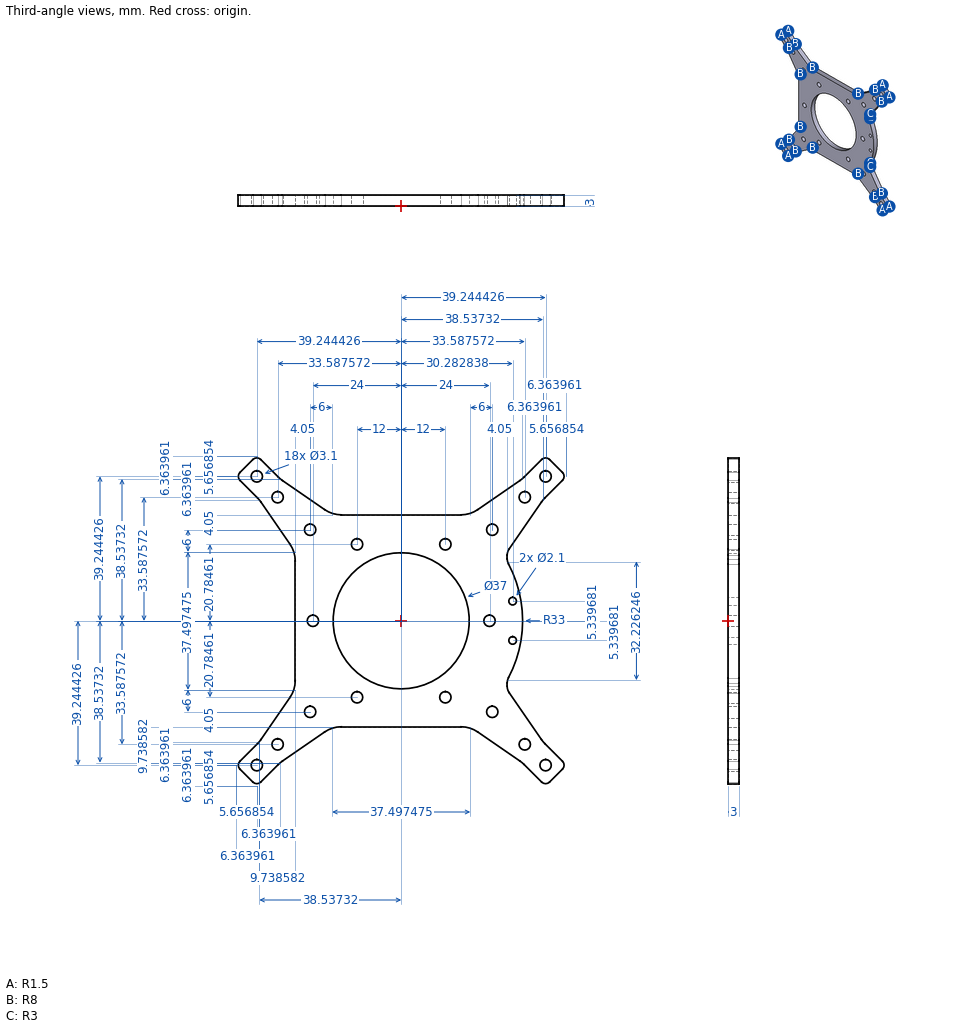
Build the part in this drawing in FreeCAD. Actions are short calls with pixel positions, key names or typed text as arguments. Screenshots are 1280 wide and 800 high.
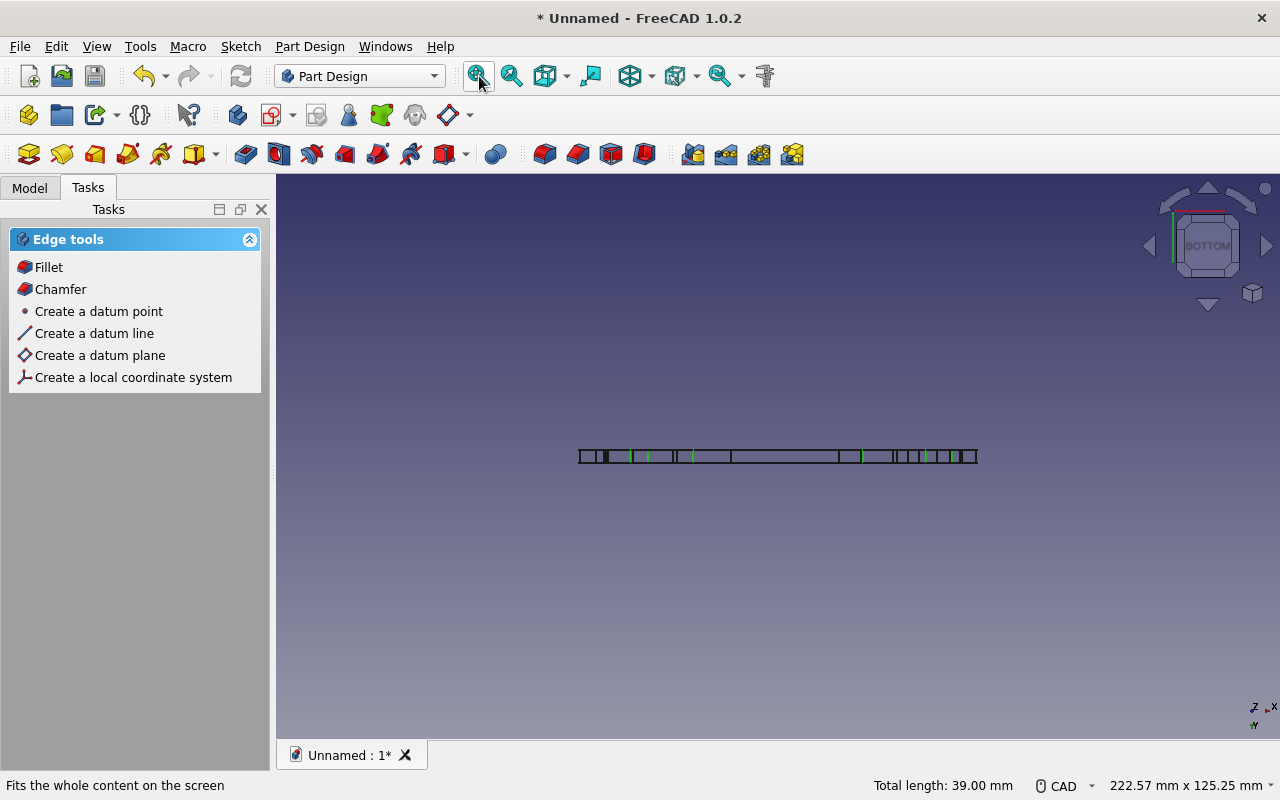
key(4)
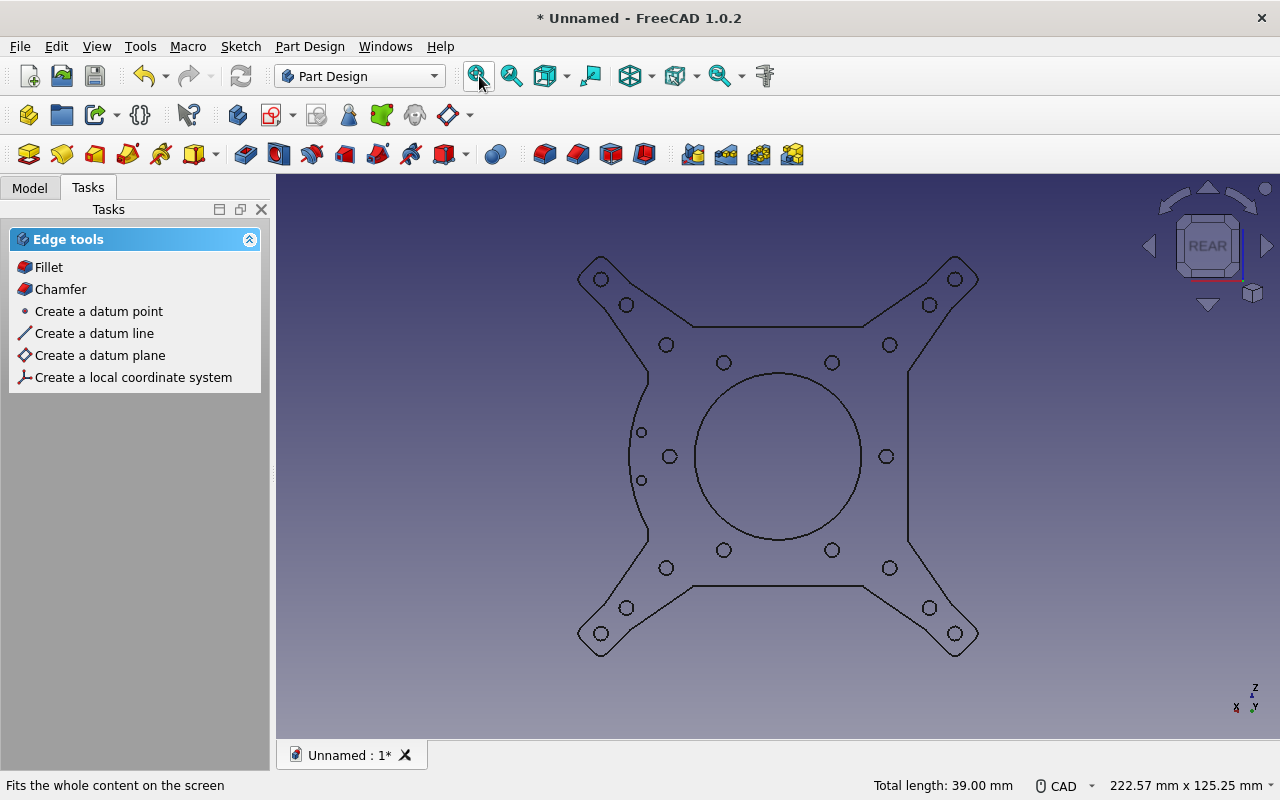
scroll(952, 604, up, 6)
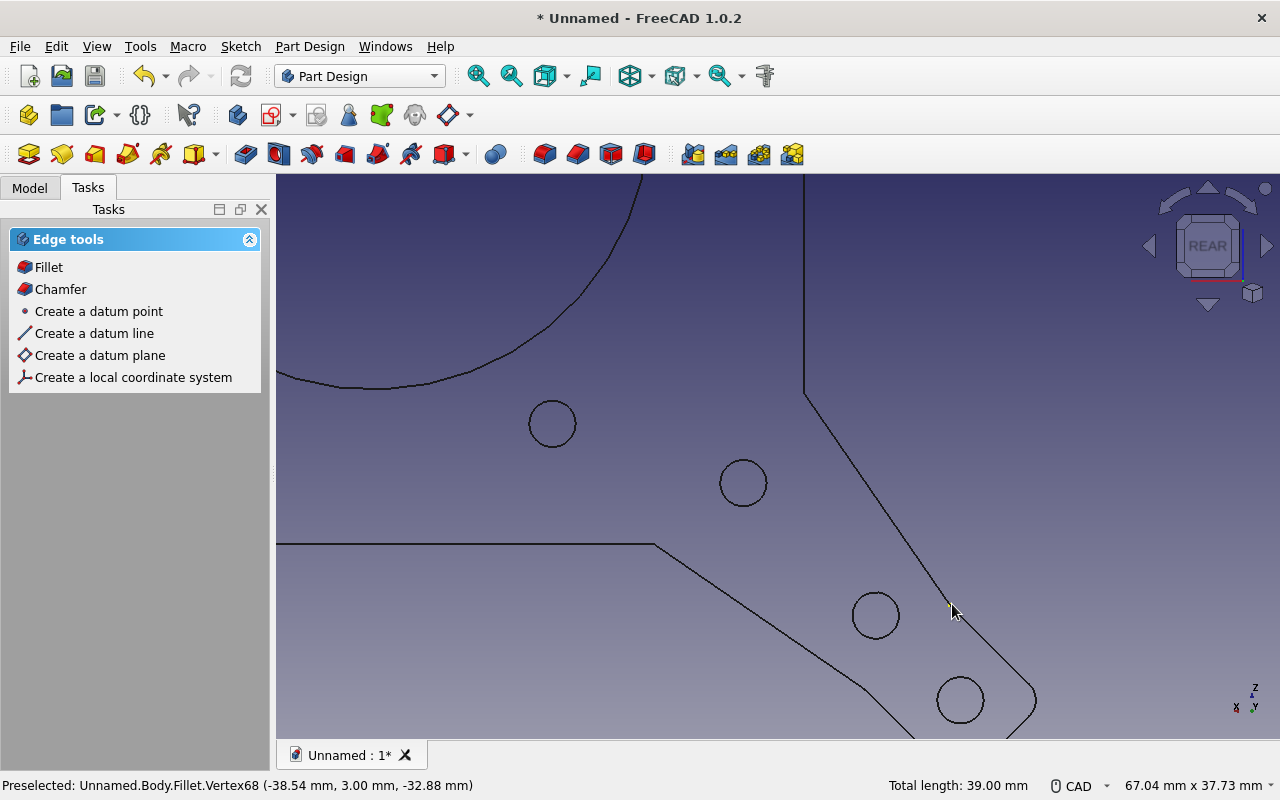
key(v)
key(f)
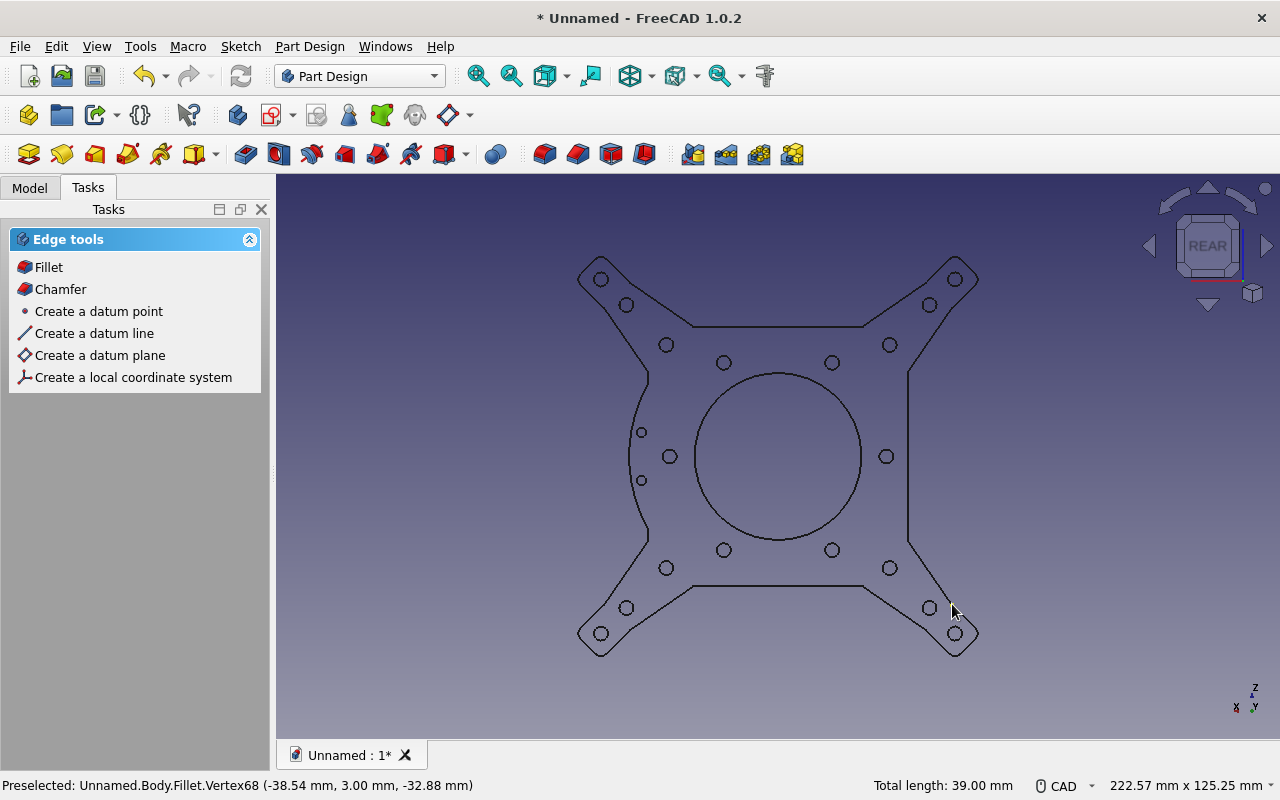
key(6)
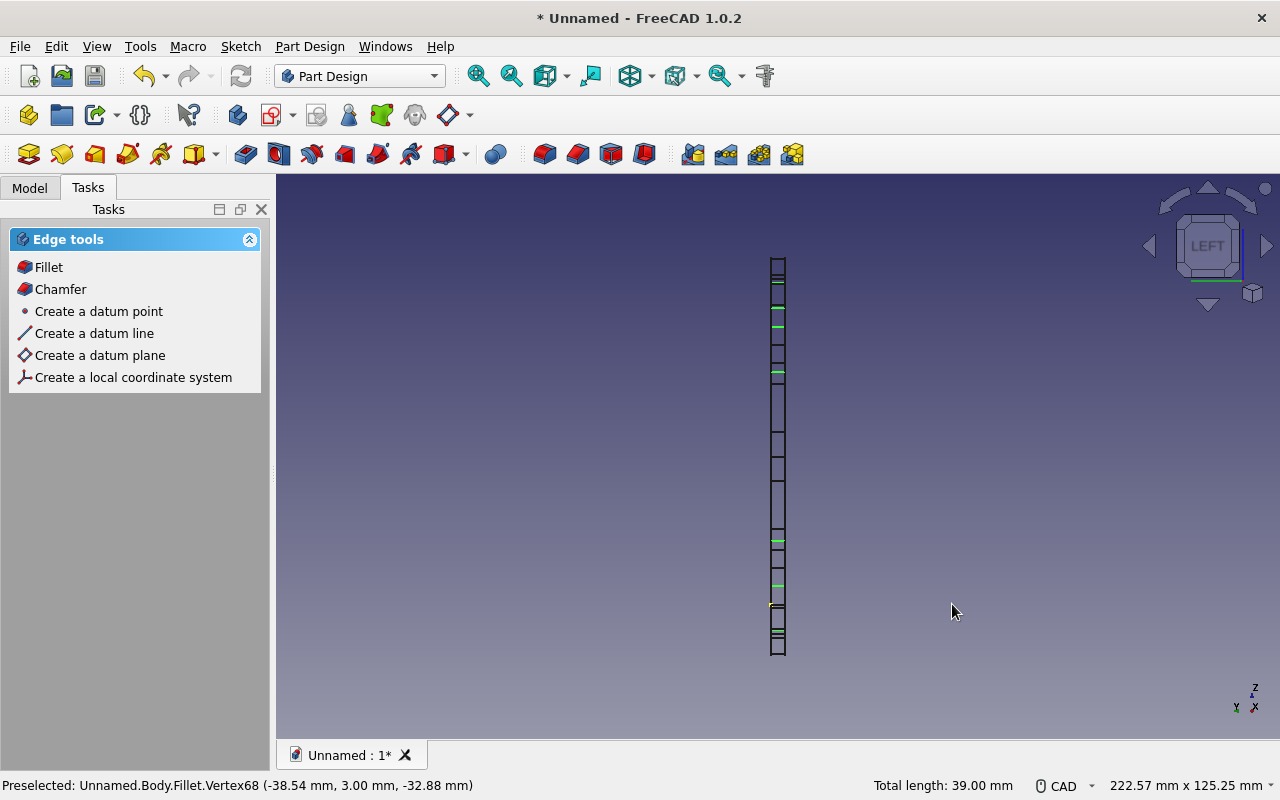
click(778, 604, ctrl)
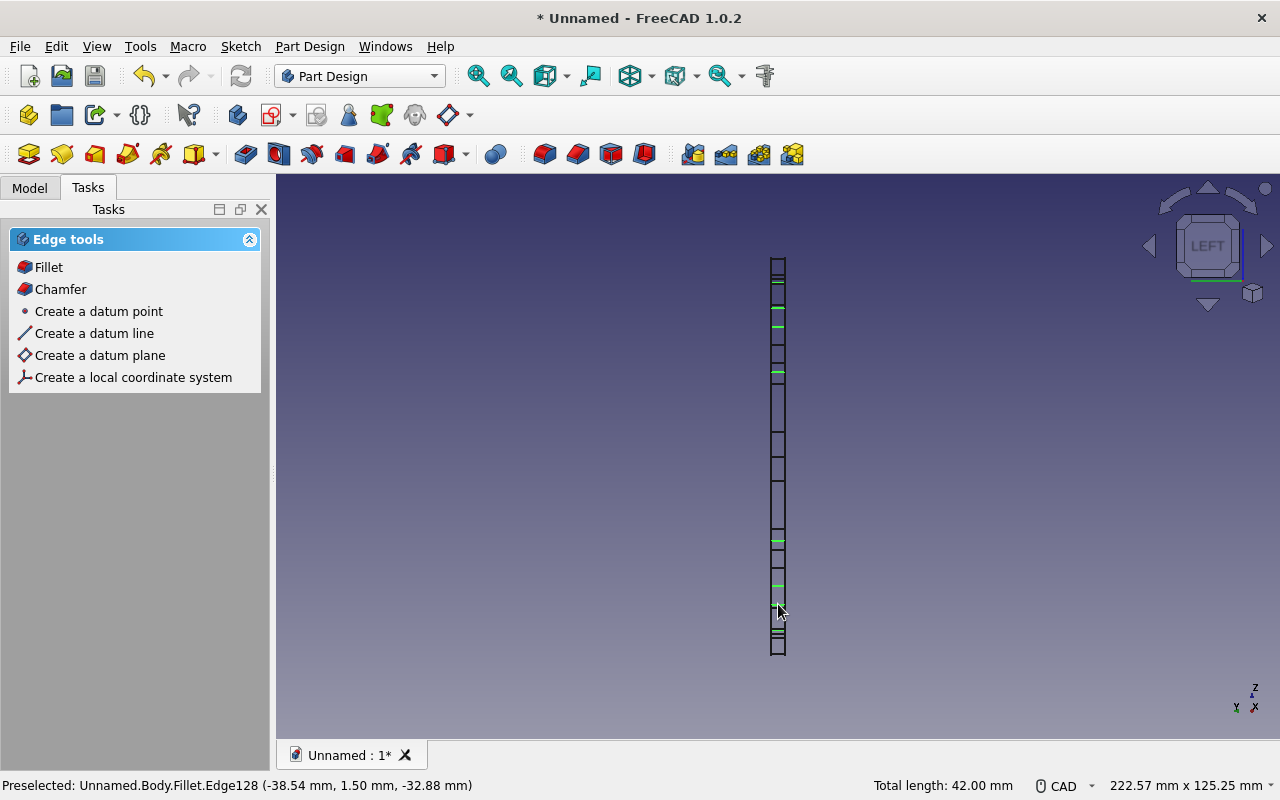
key(v)
key(1)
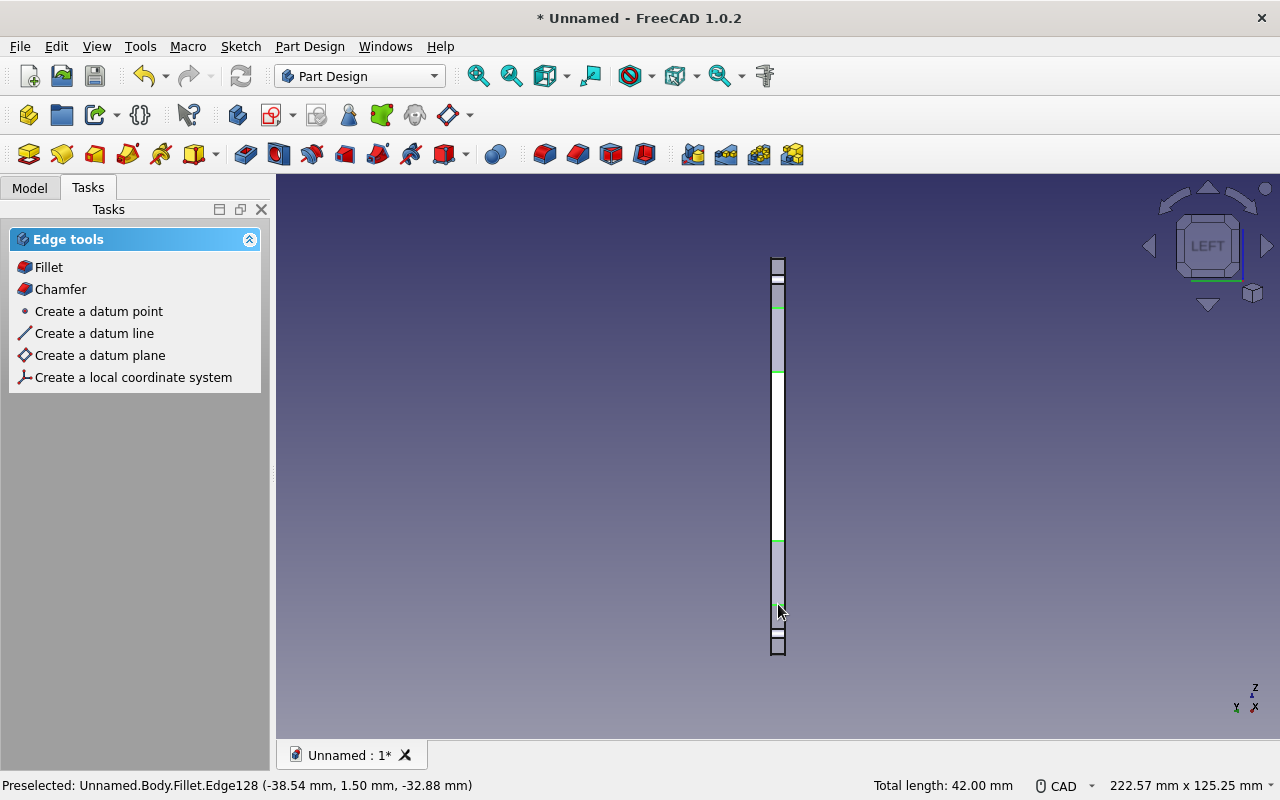
click(545, 154)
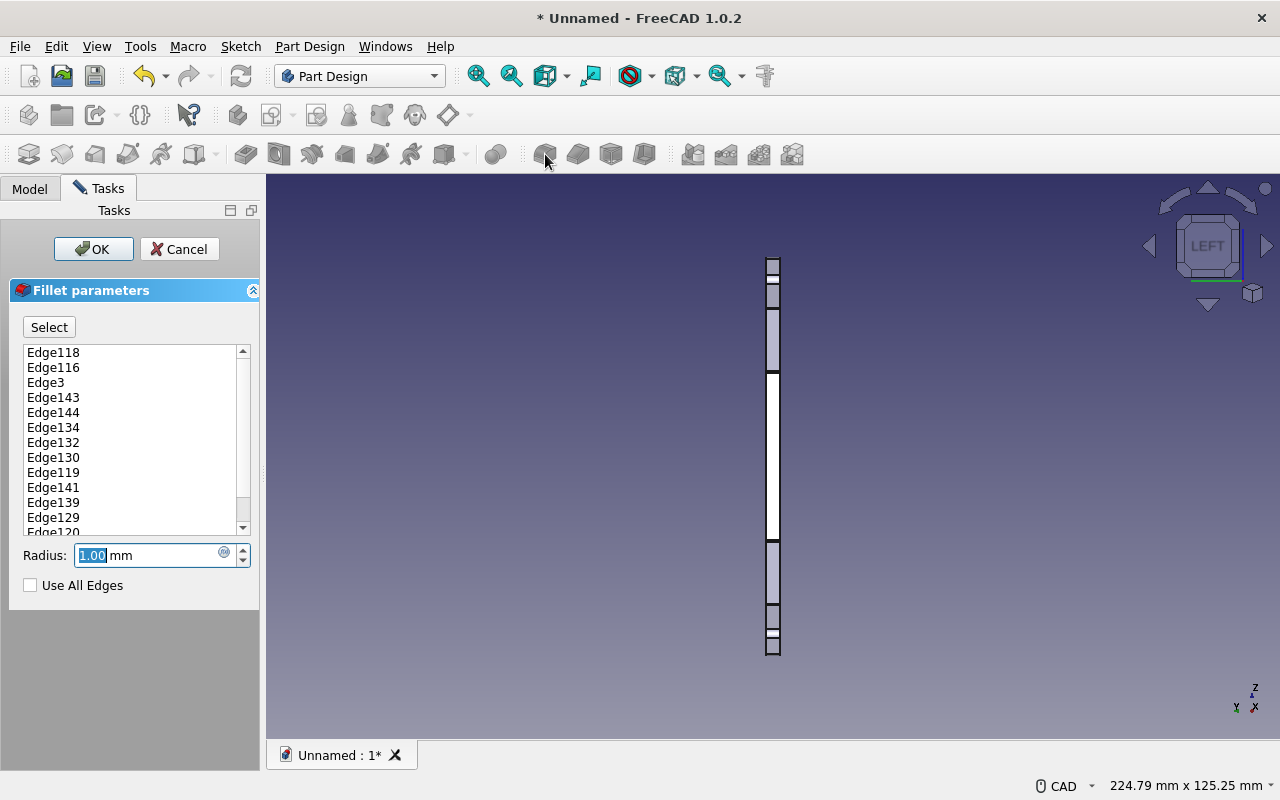
text(8)
key(Tab)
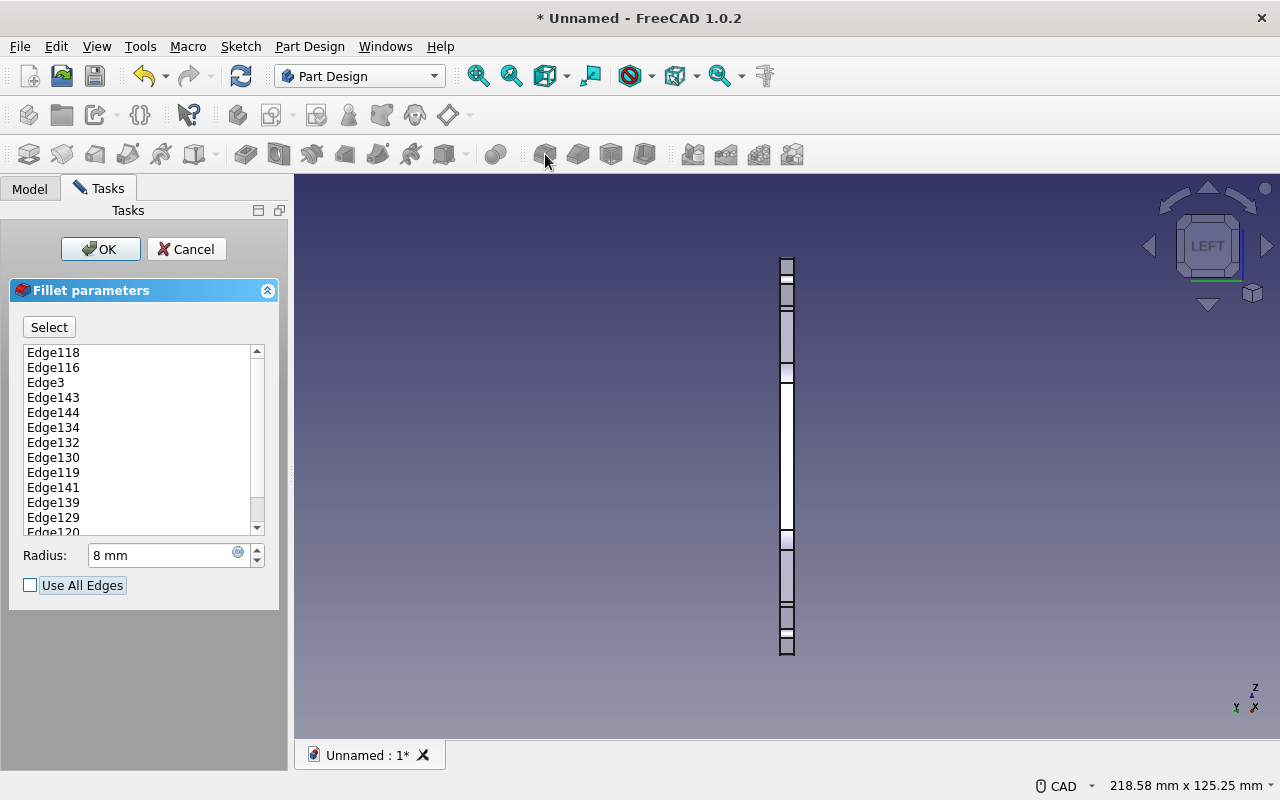
click(101, 249)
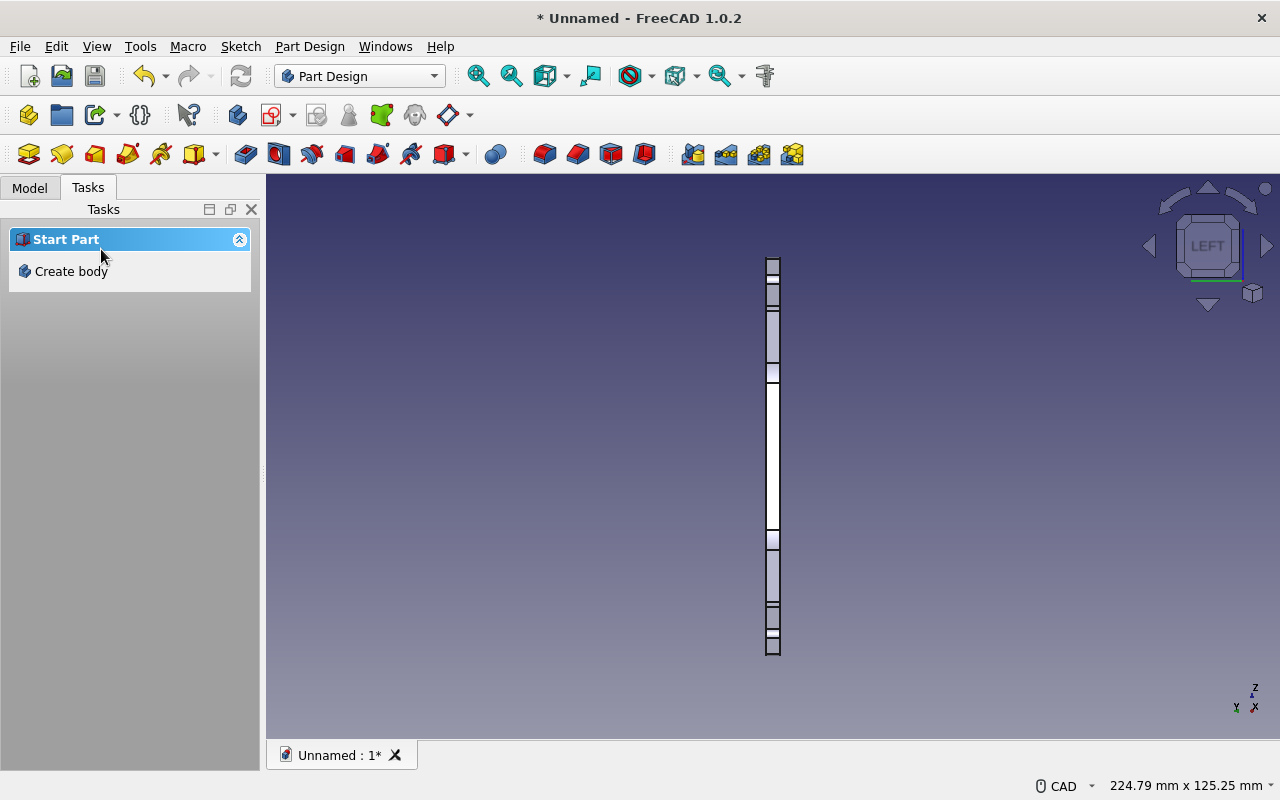
scroll(773, 383, up, 6)